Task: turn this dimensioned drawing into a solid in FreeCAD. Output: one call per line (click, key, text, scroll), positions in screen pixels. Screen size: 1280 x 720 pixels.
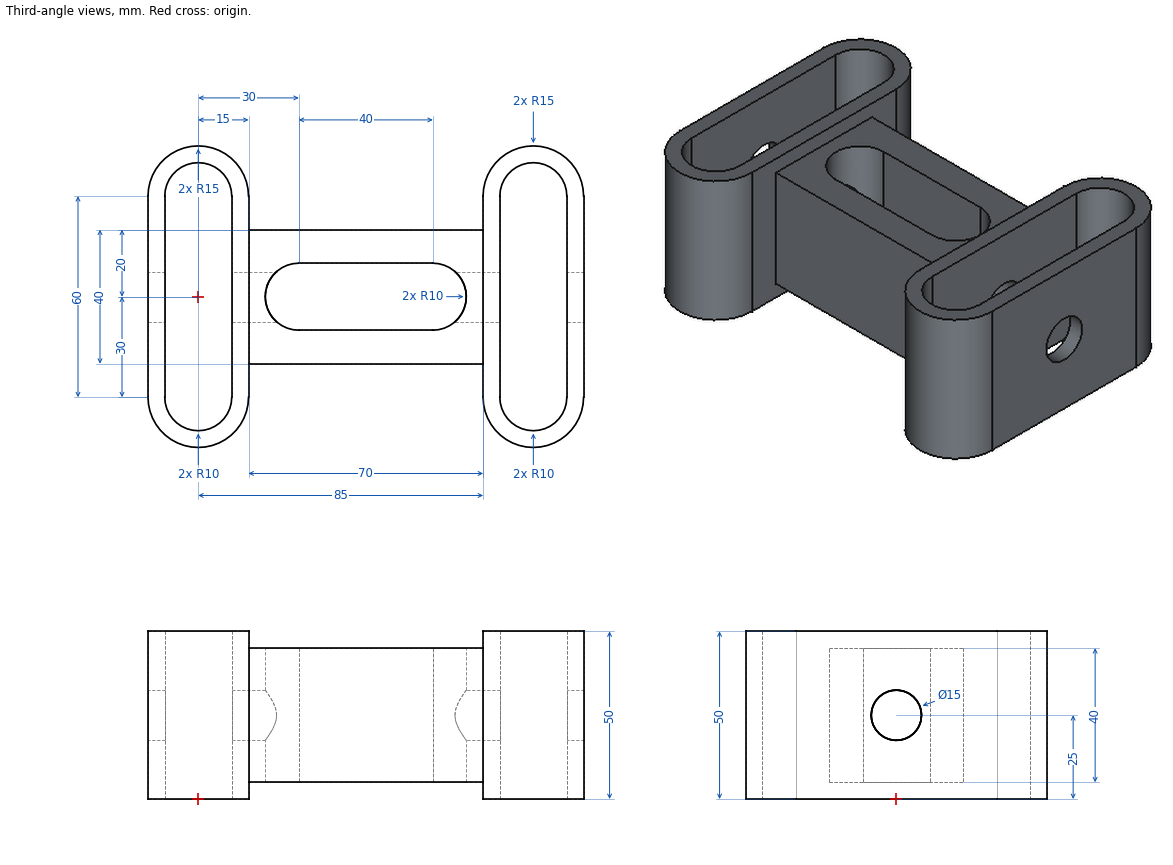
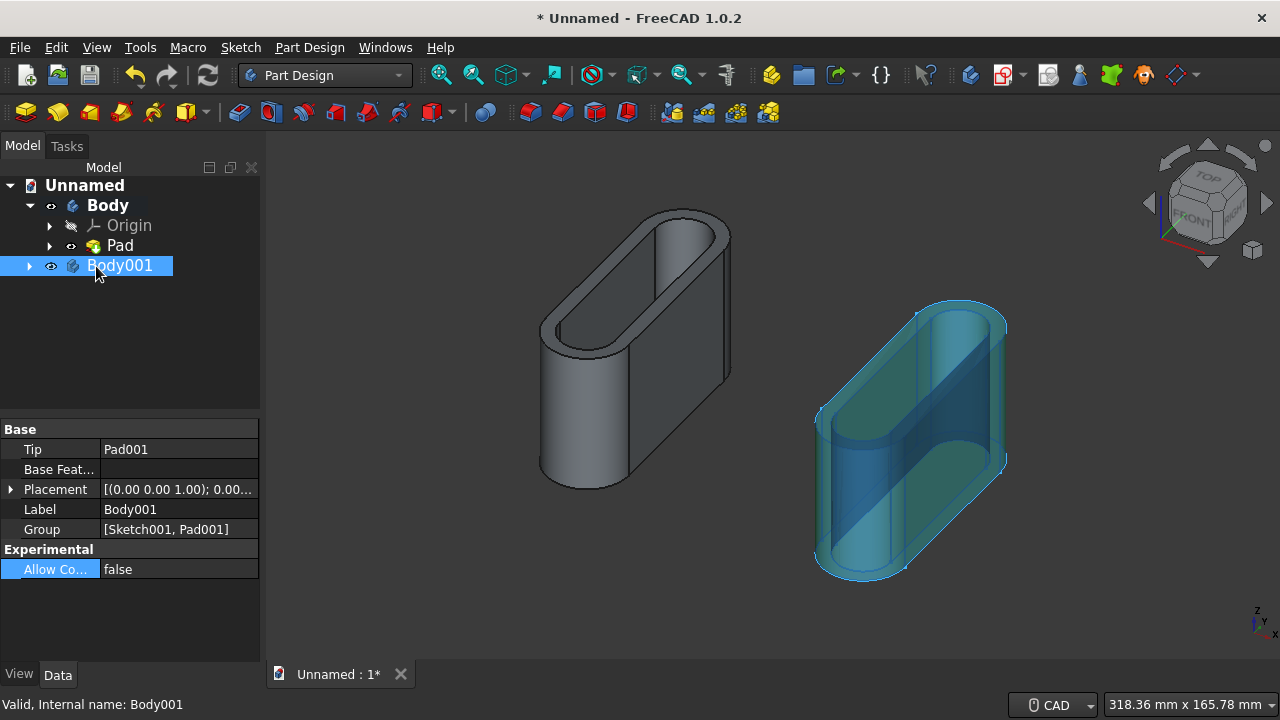
click(486, 112)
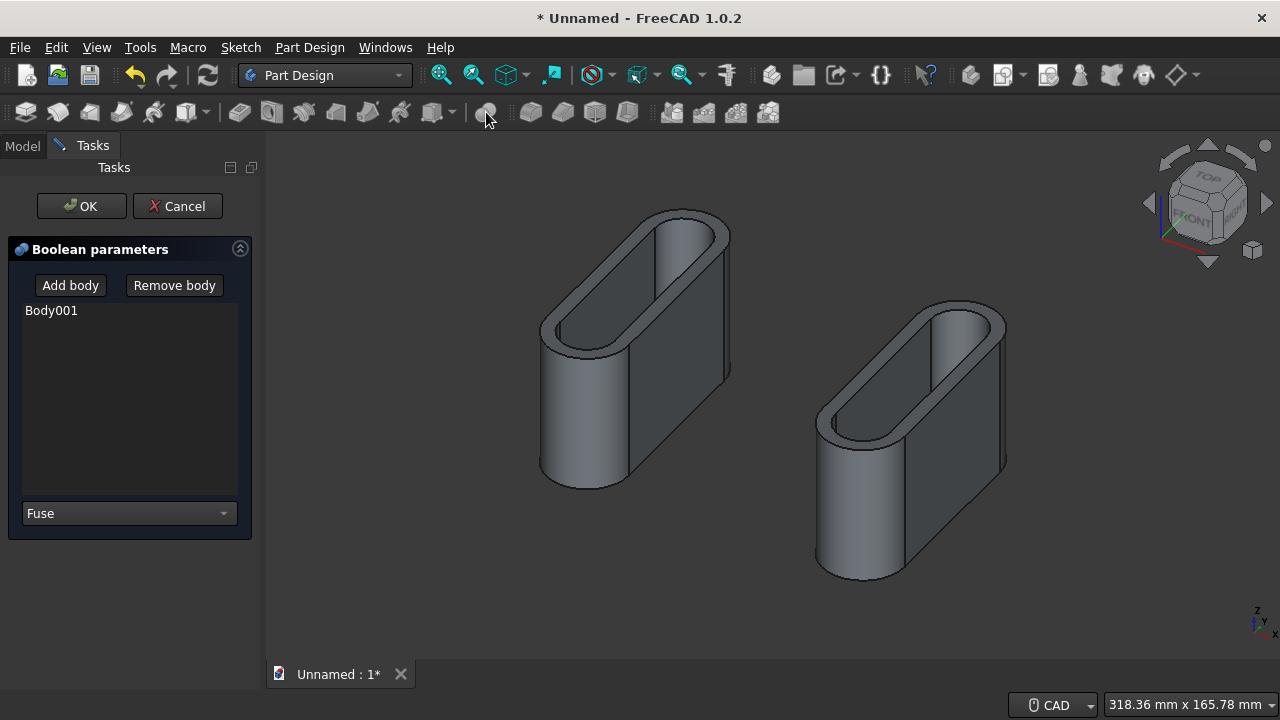
click(82, 206)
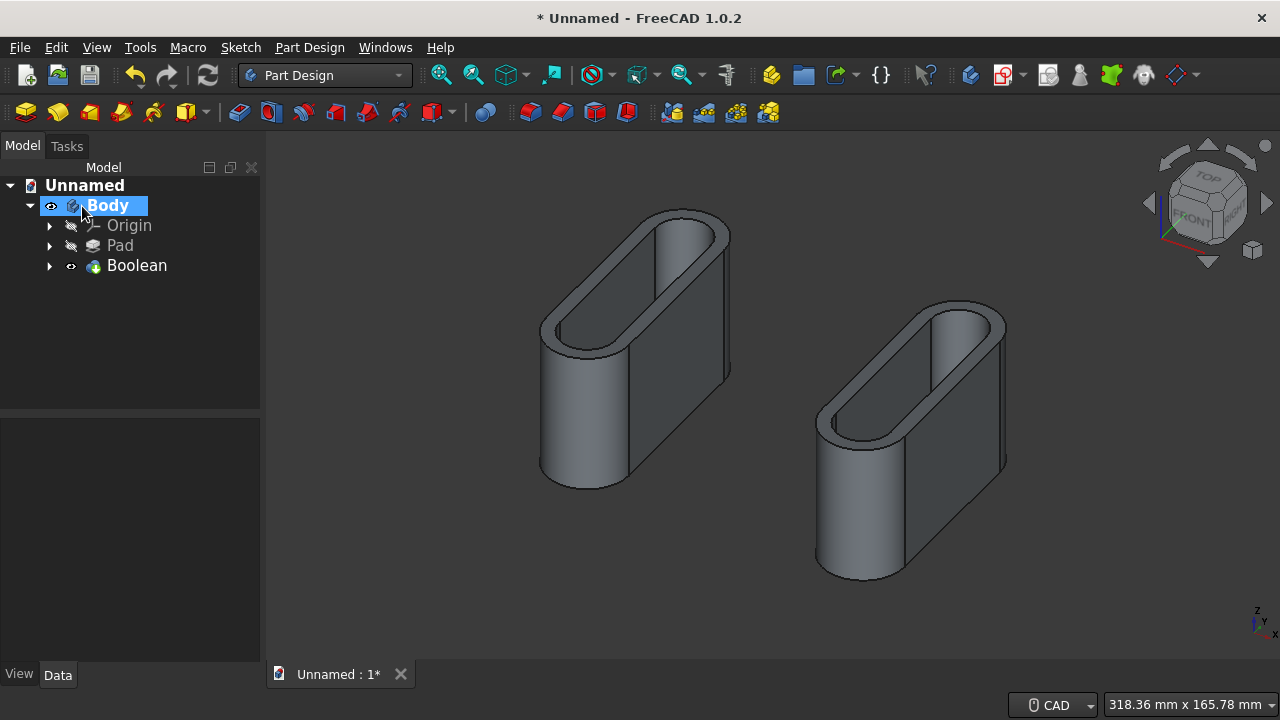
click(50, 226)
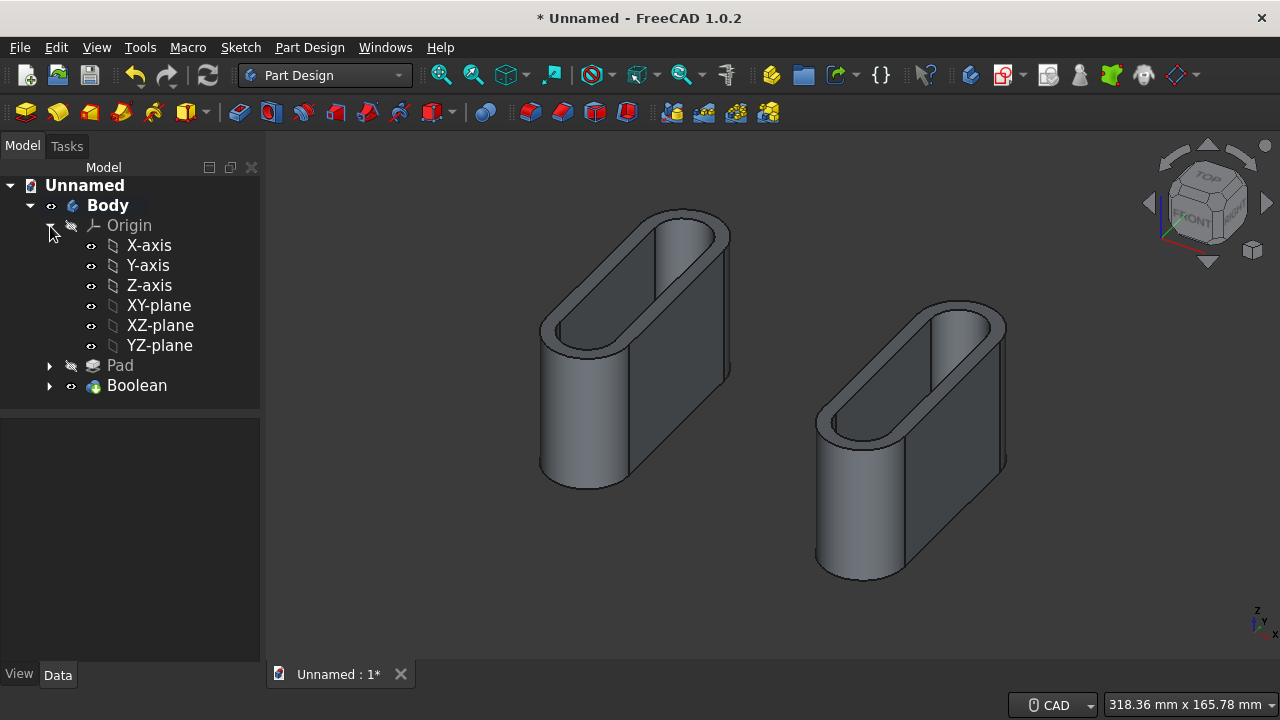
click(136, 306)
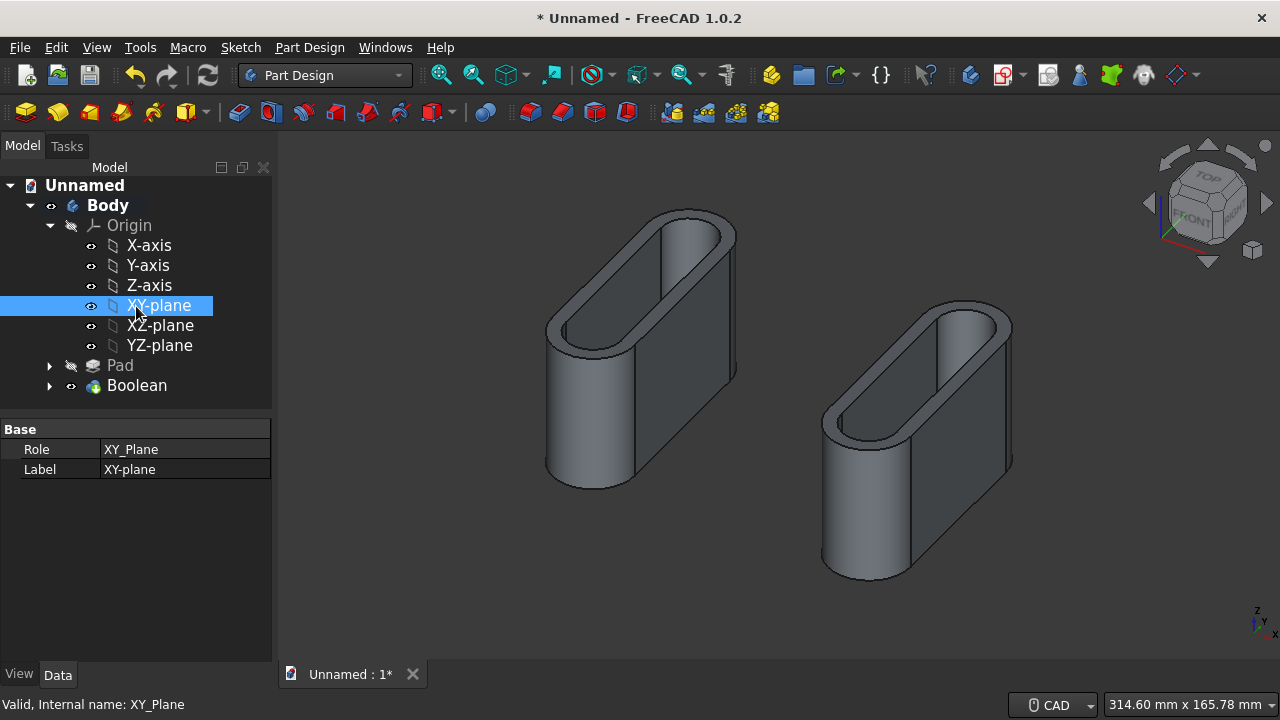
click(1176, 76)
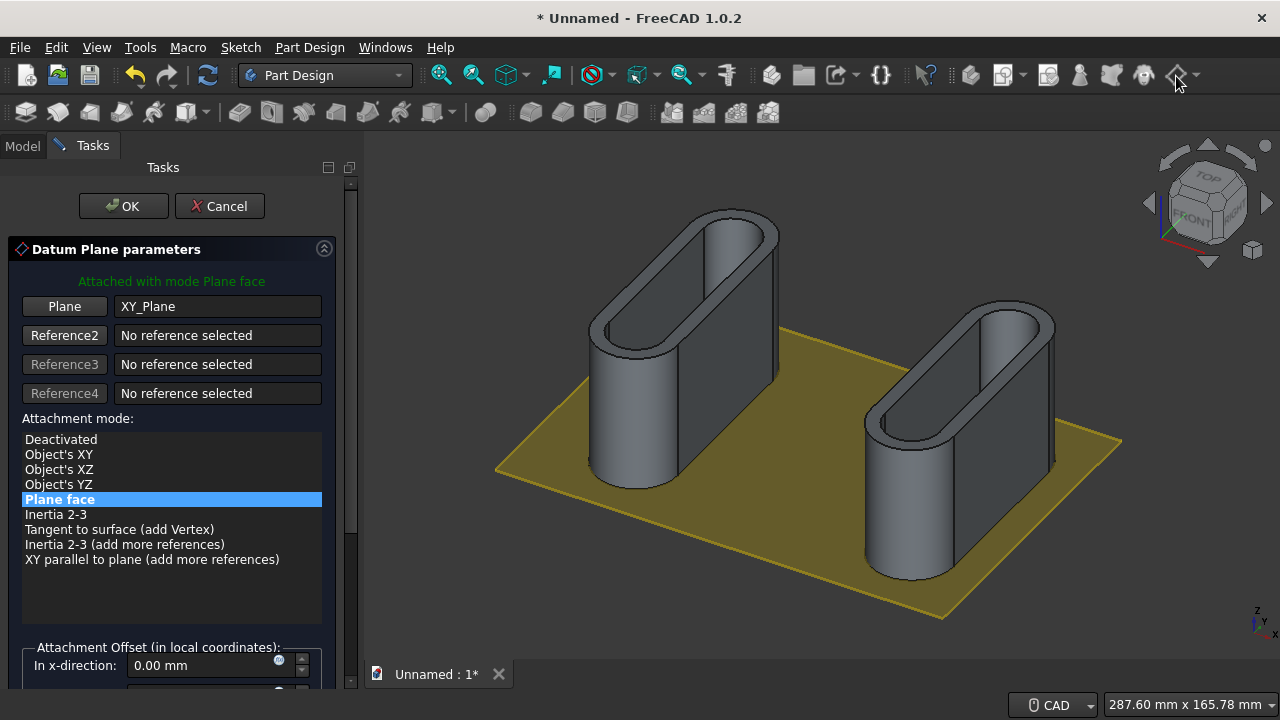
scroll(351, 432, down, 2)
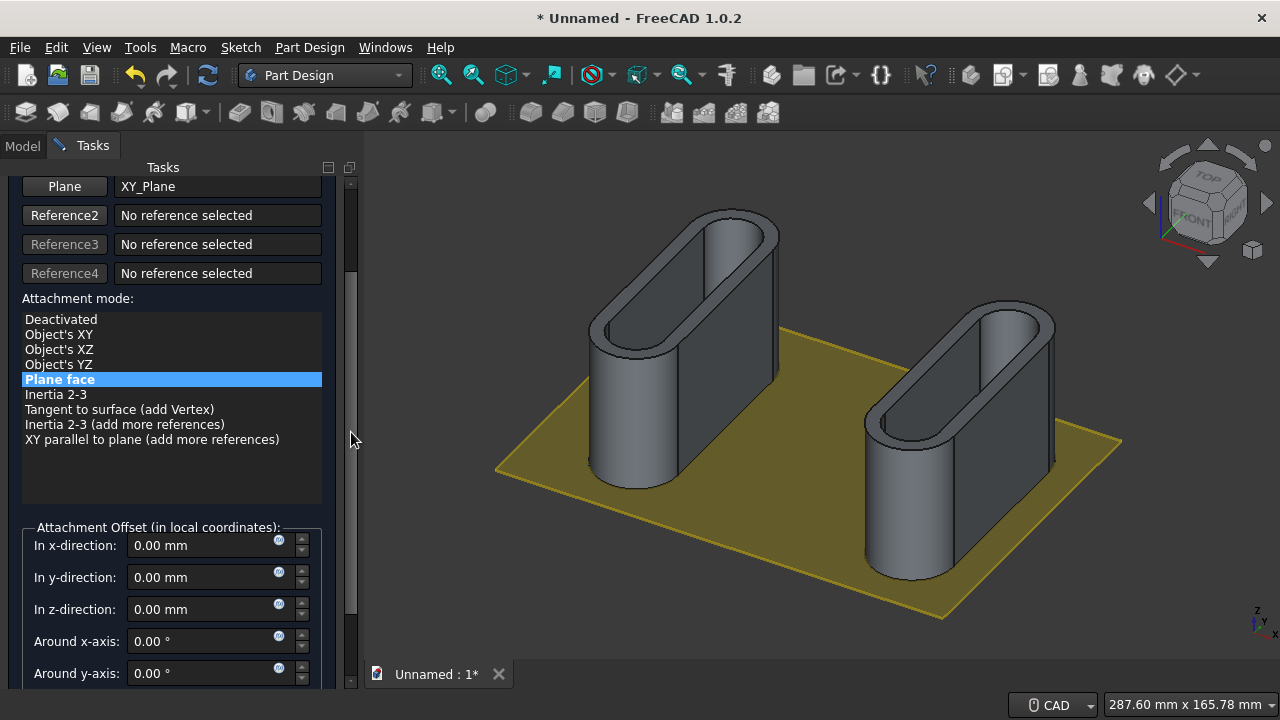
triple_click(210, 609)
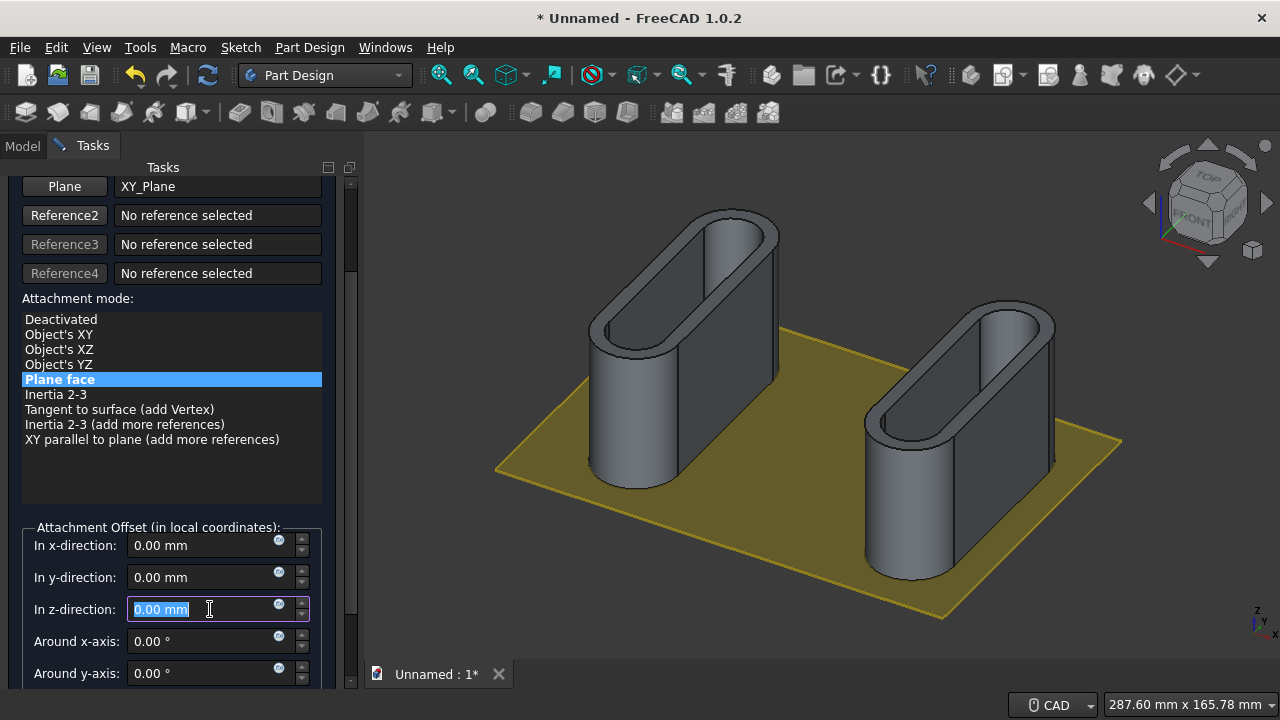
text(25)
key(Tab)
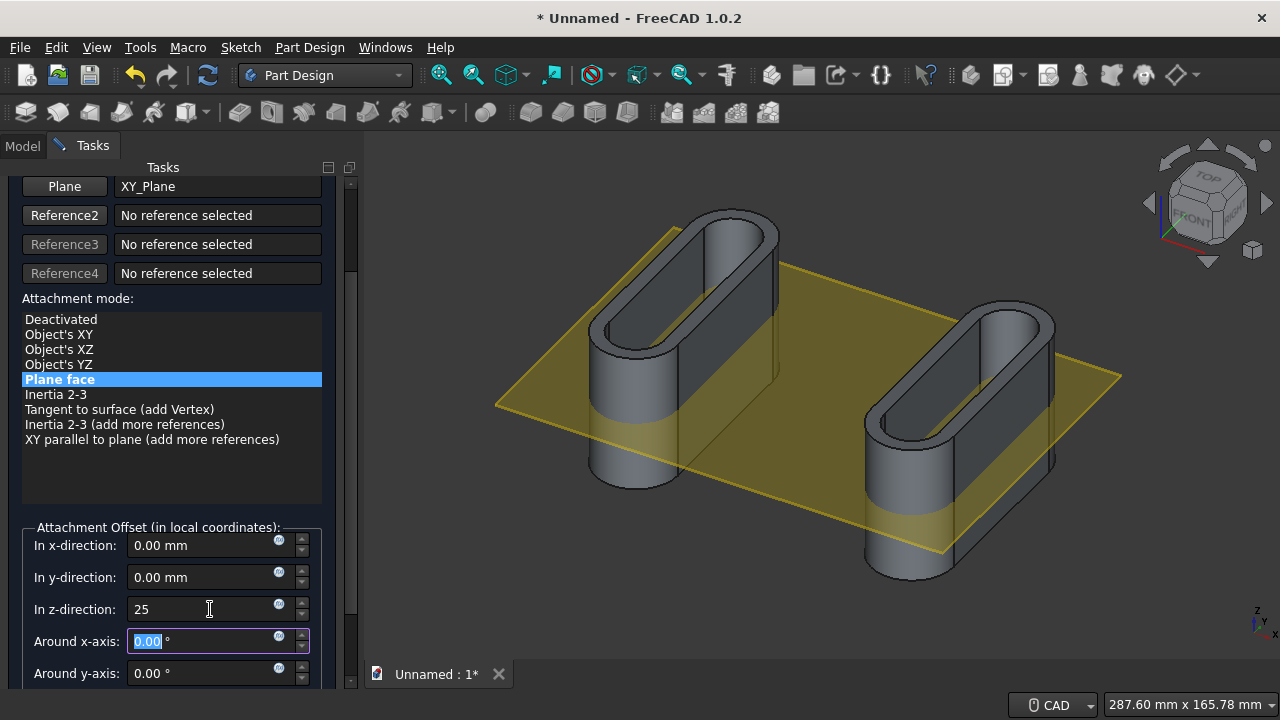
scroll(351, 432, up, 3)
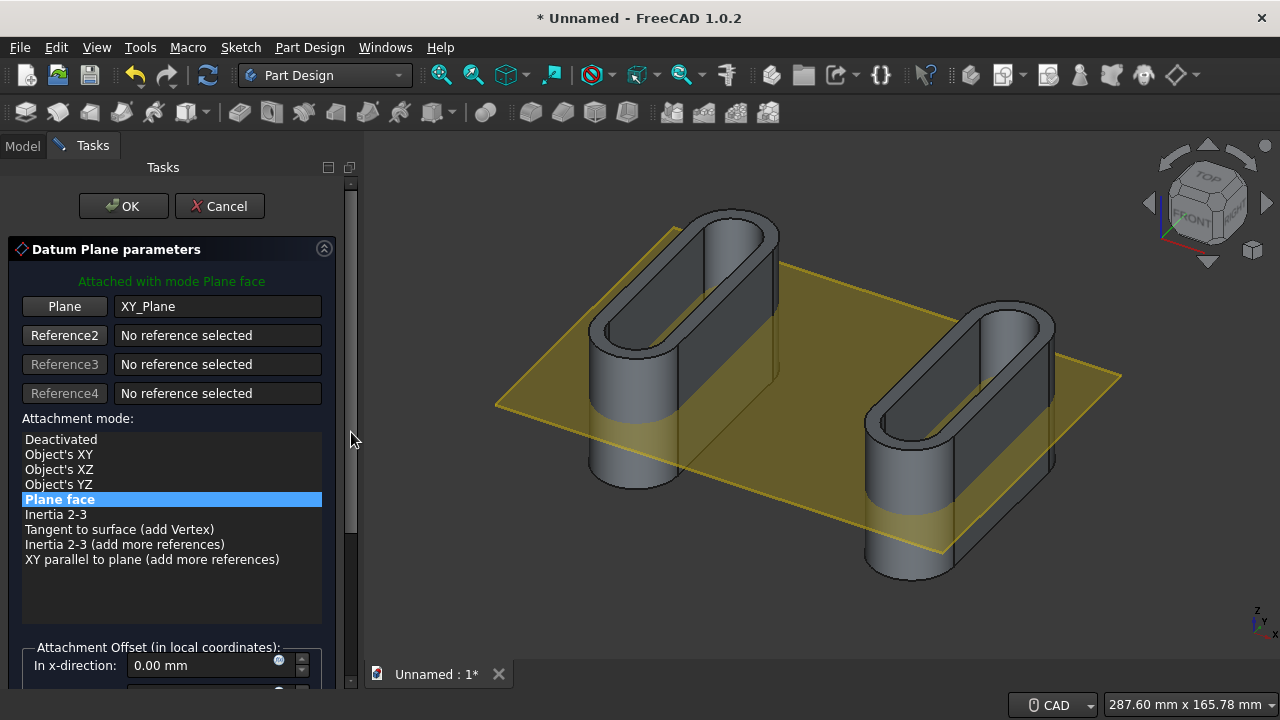
click(124, 206)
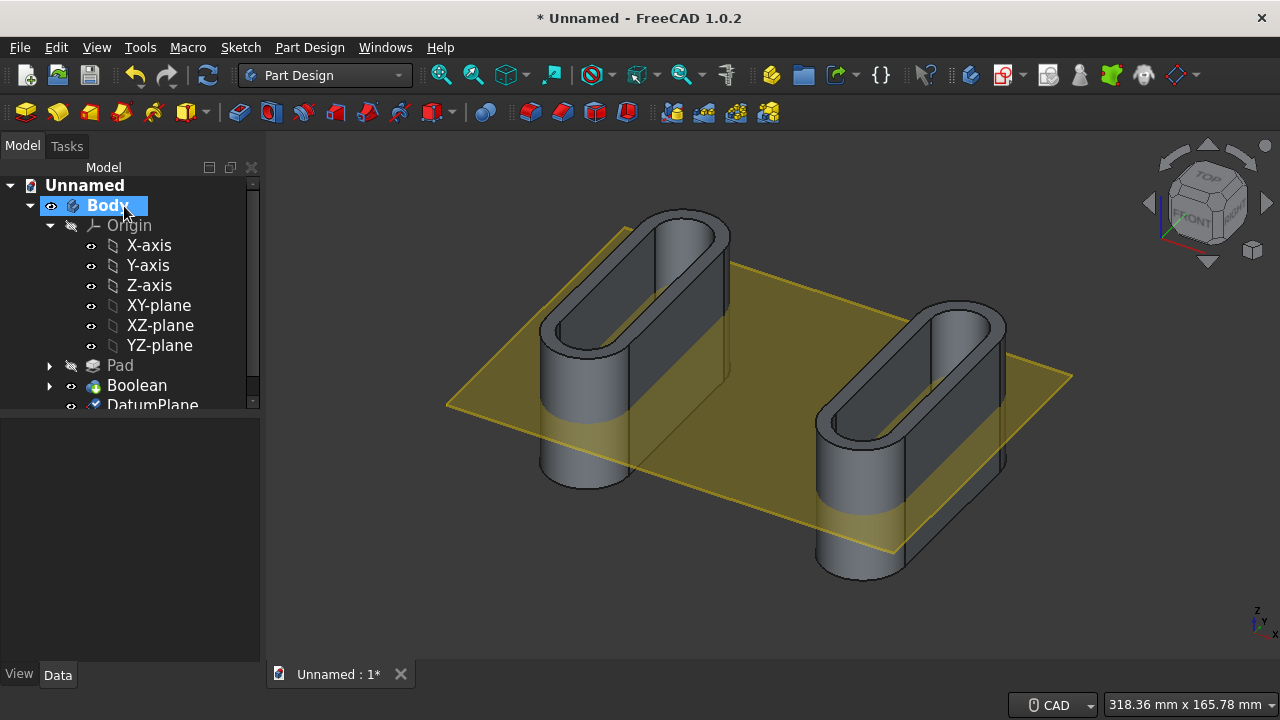
click(116, 406)